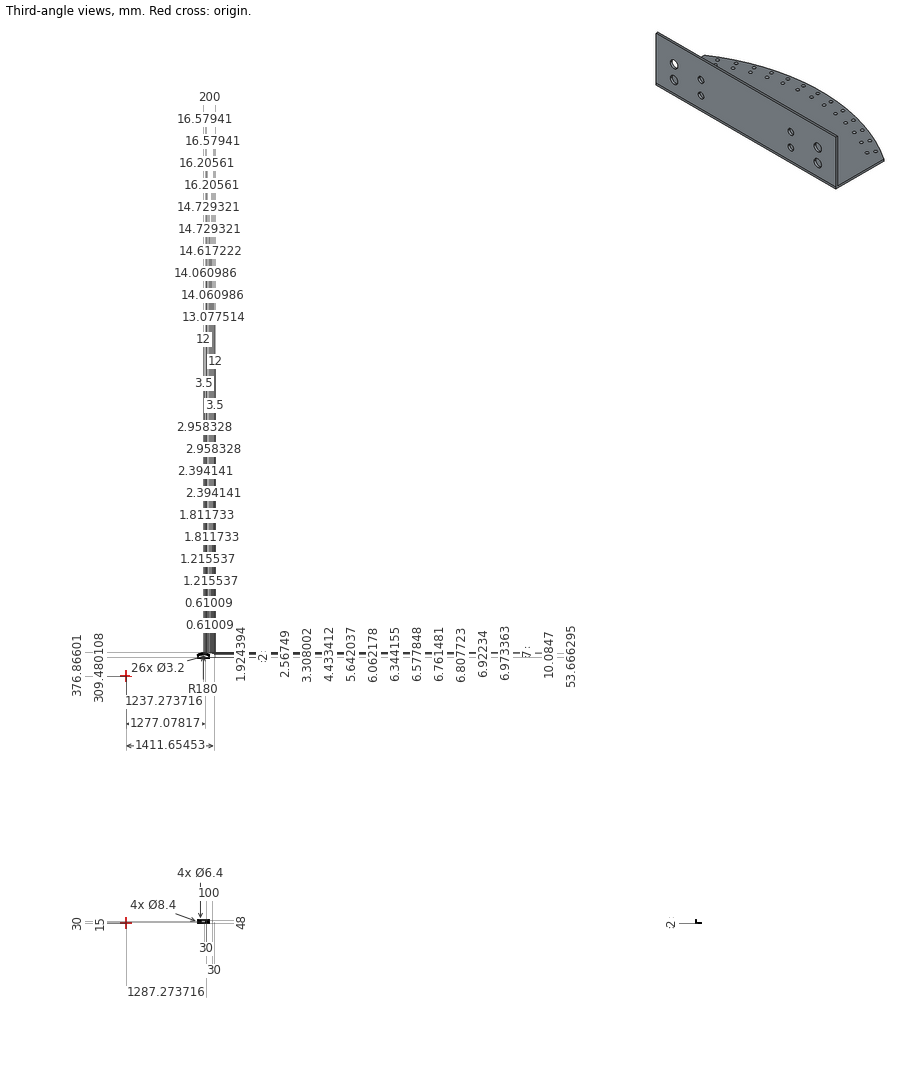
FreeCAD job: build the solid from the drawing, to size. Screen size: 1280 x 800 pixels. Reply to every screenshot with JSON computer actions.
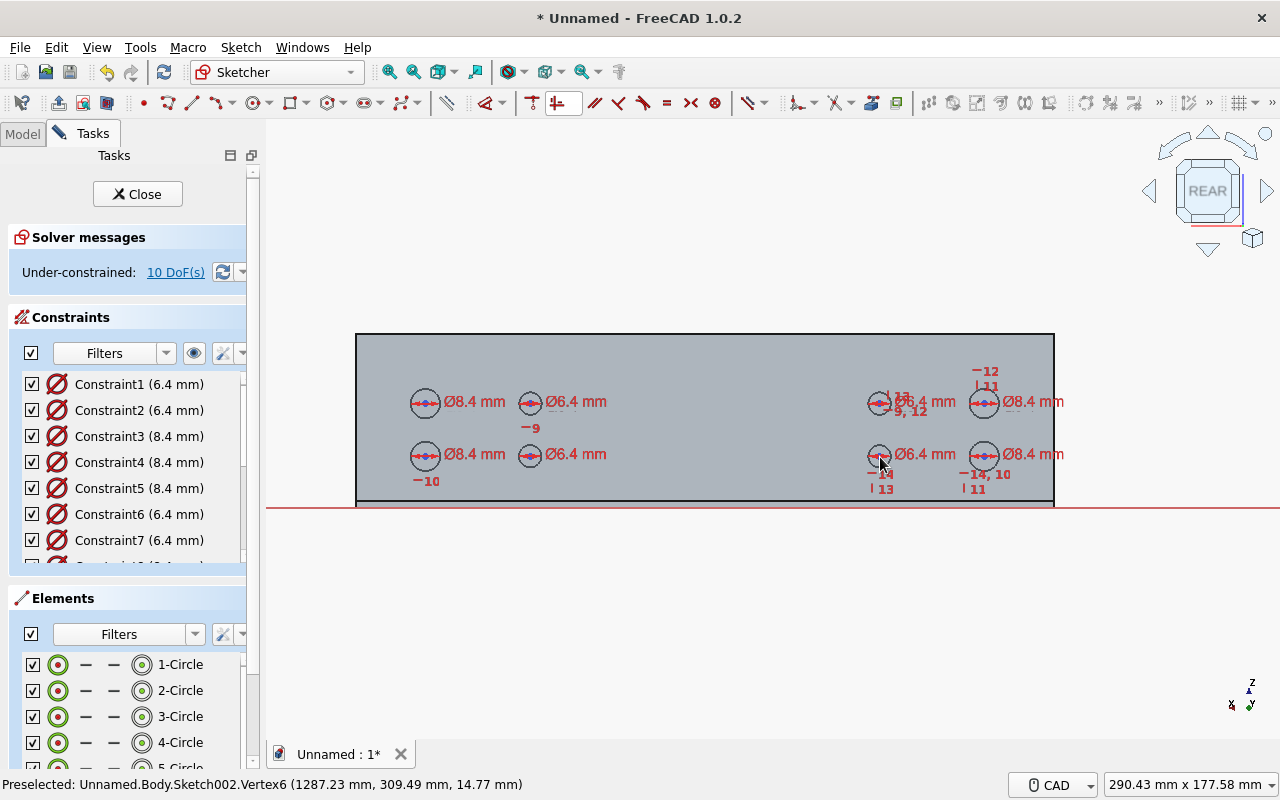
{"action": "left_click", "coordinate": [530, 404]}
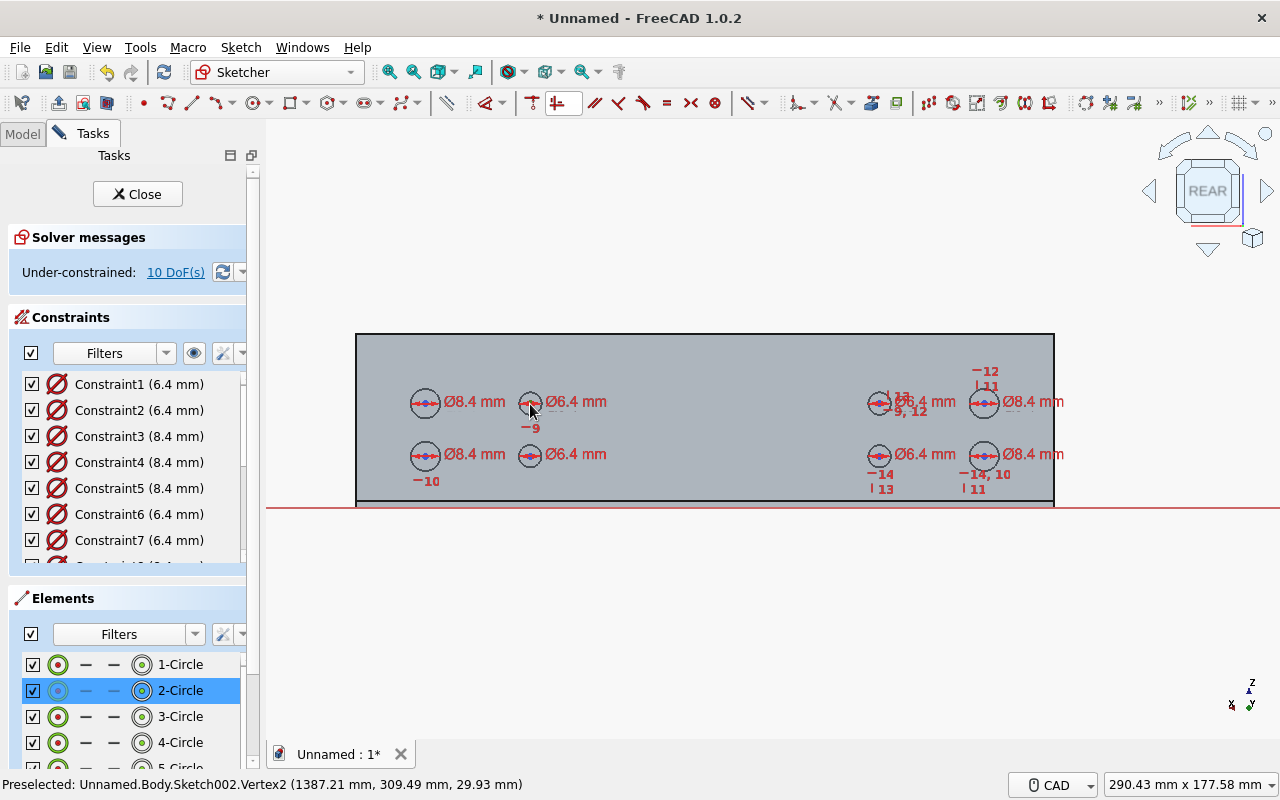
{"action": "left_click", "coordinate": [530, 456]}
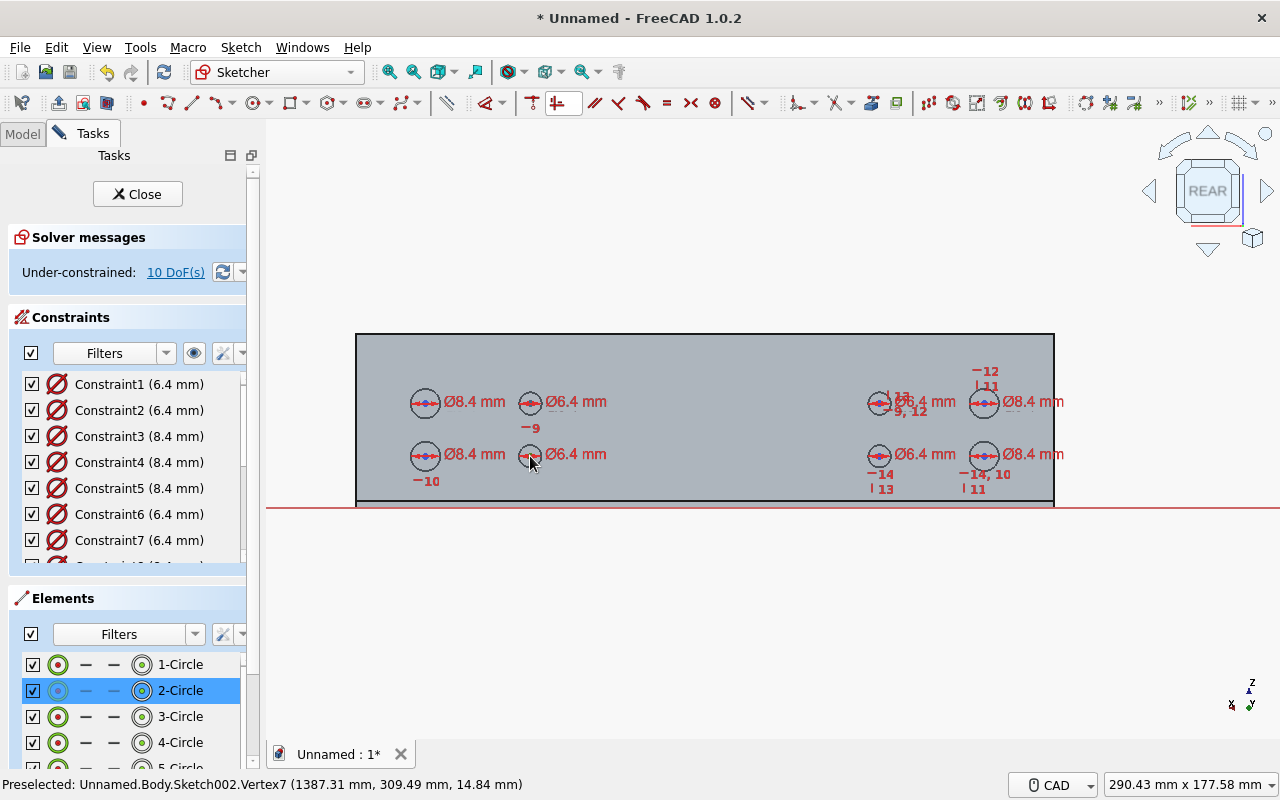
{"action": "key", "text": "v"}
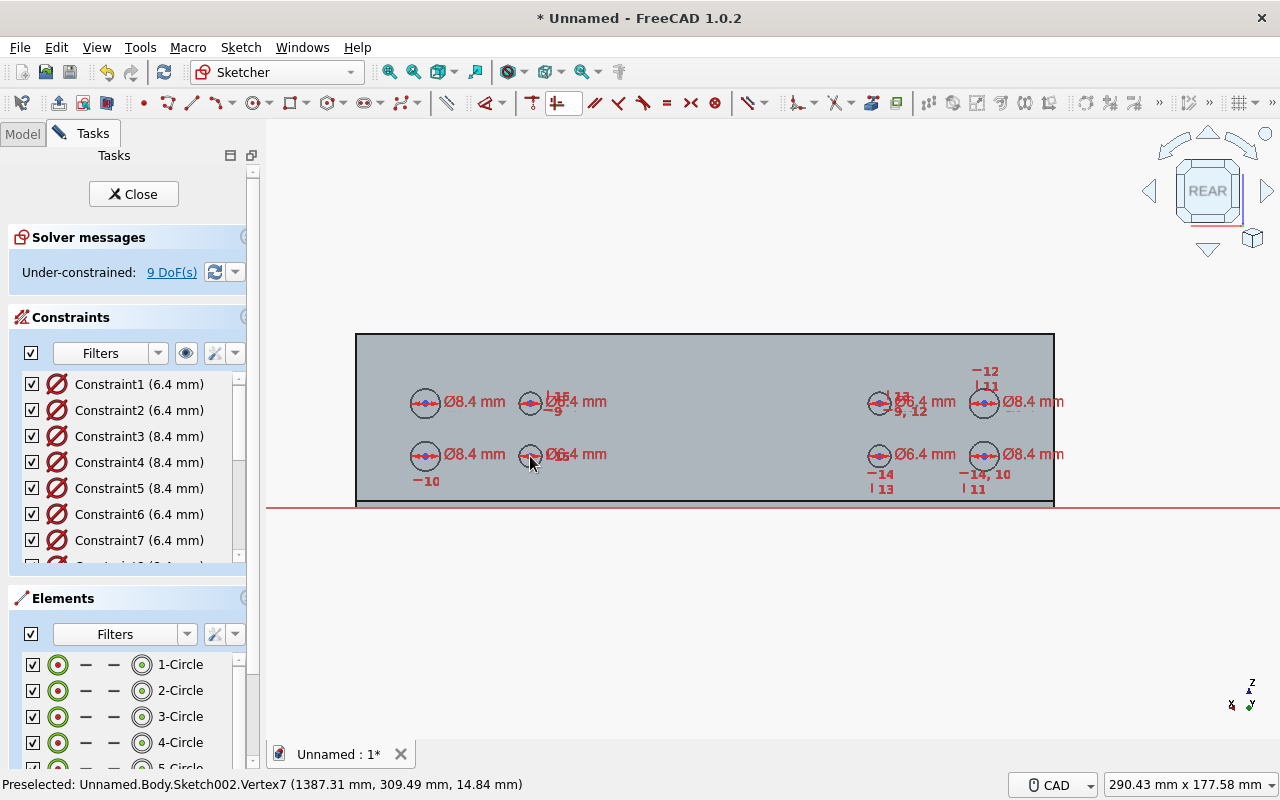
{"action": "left_click", "coordinate": [426, 456]}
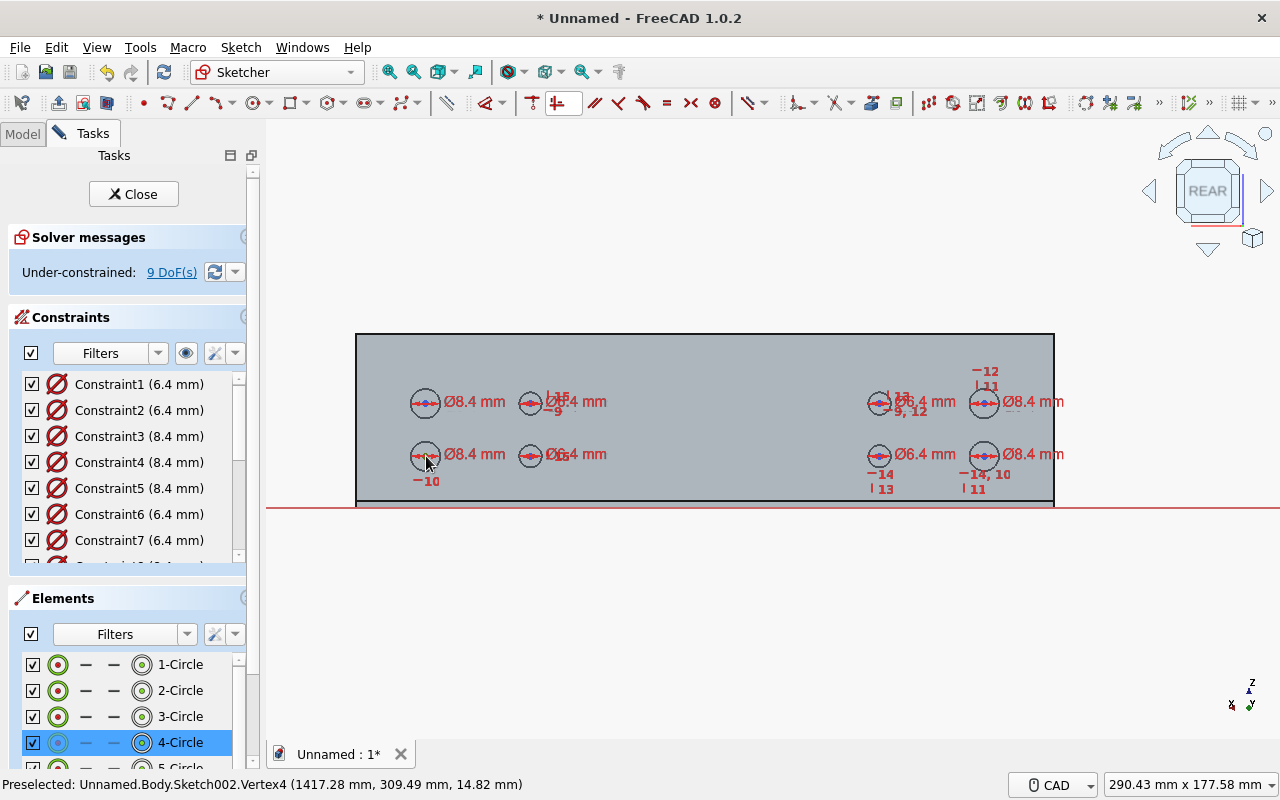
{"action": "left_click", "coordinate": [530, 456]}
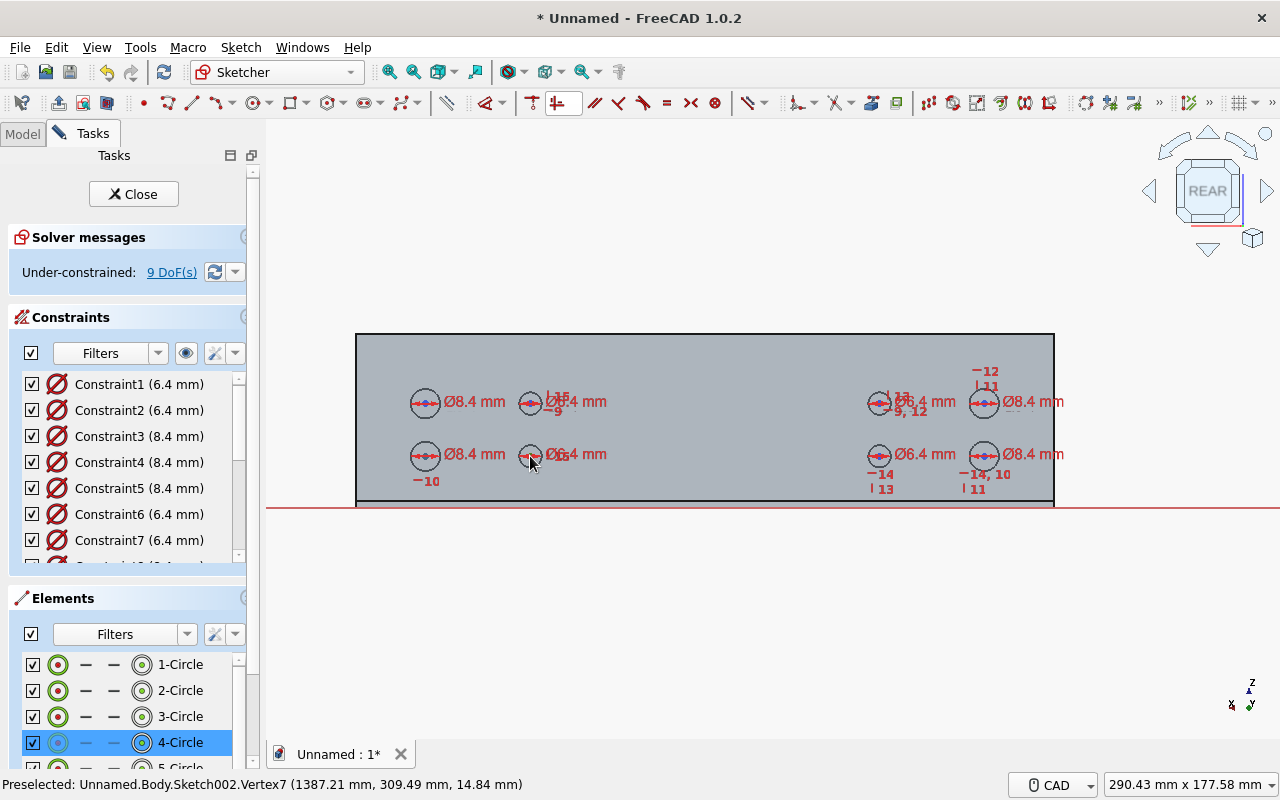
{"action": "key", "text": "h"}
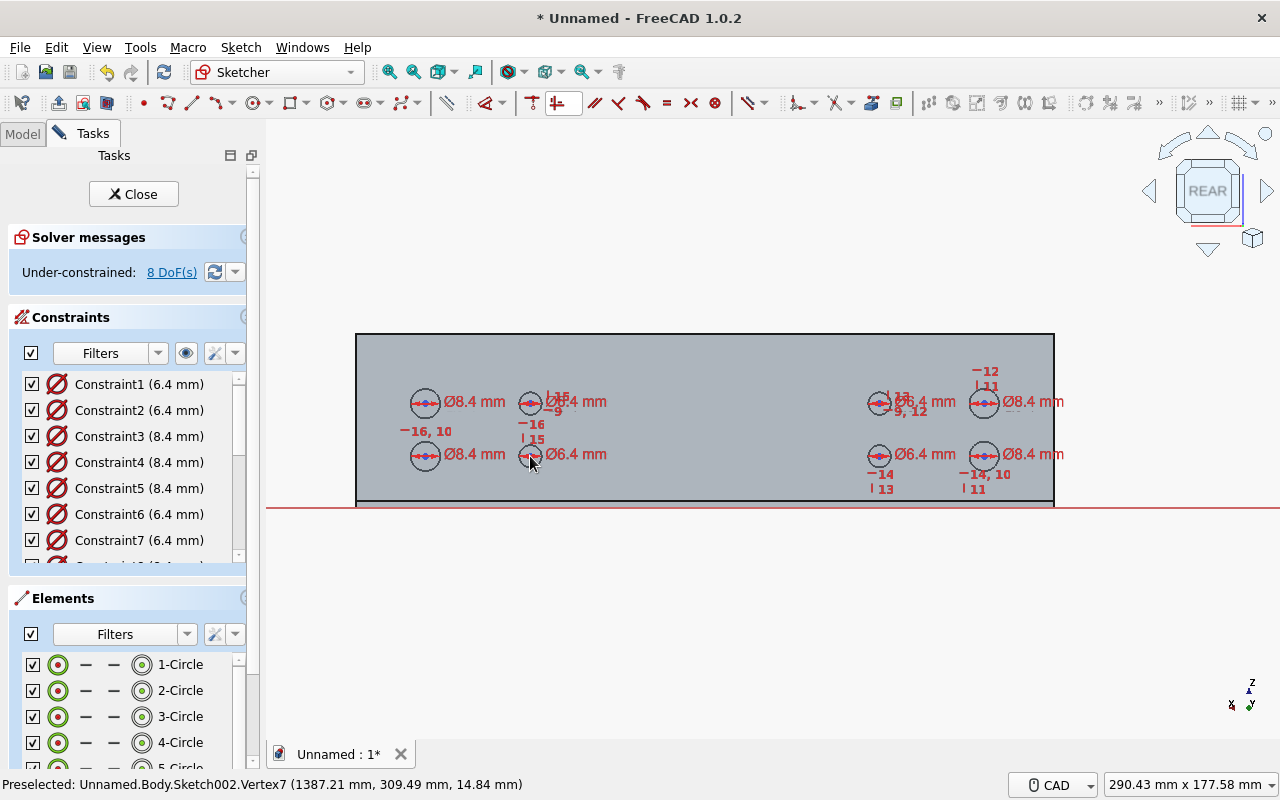
{"action": "left_click", "coordinate": [426, 456]}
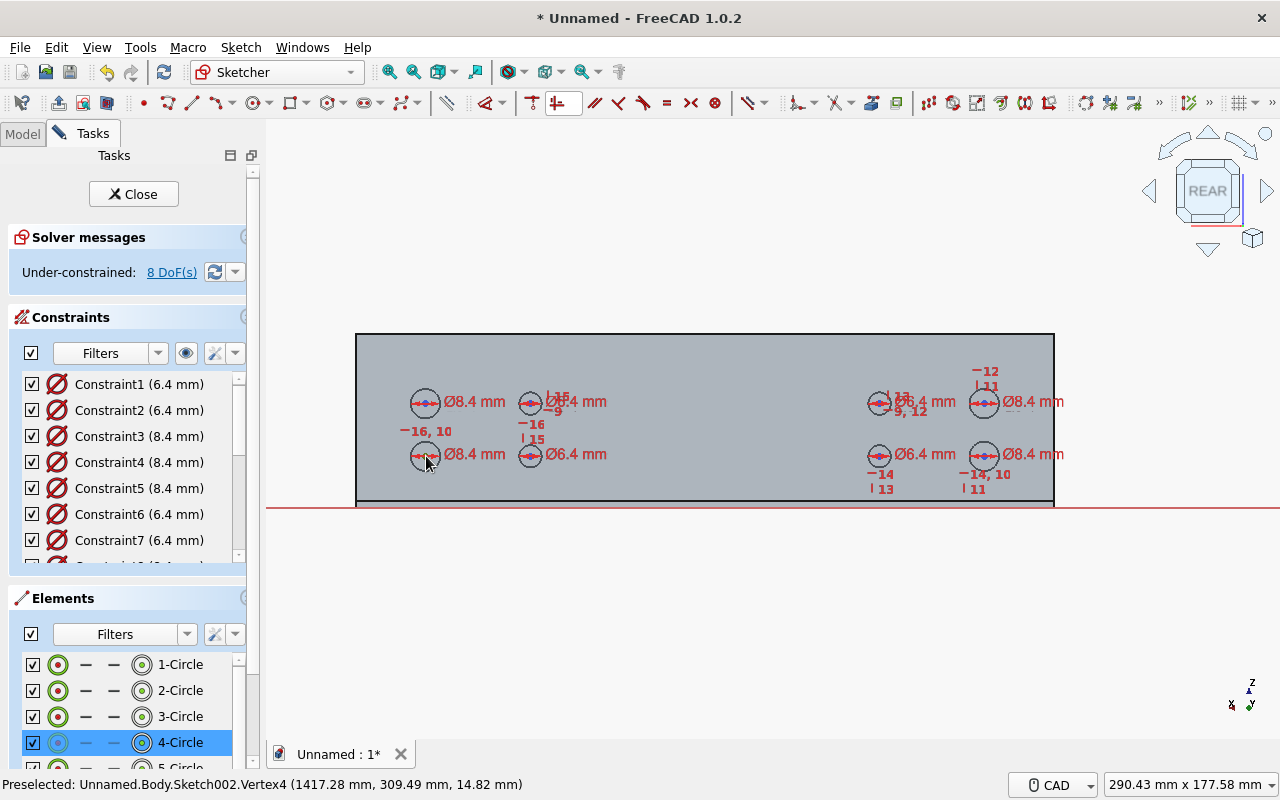
{"action": "left_click", "coordinate": [425, 404]}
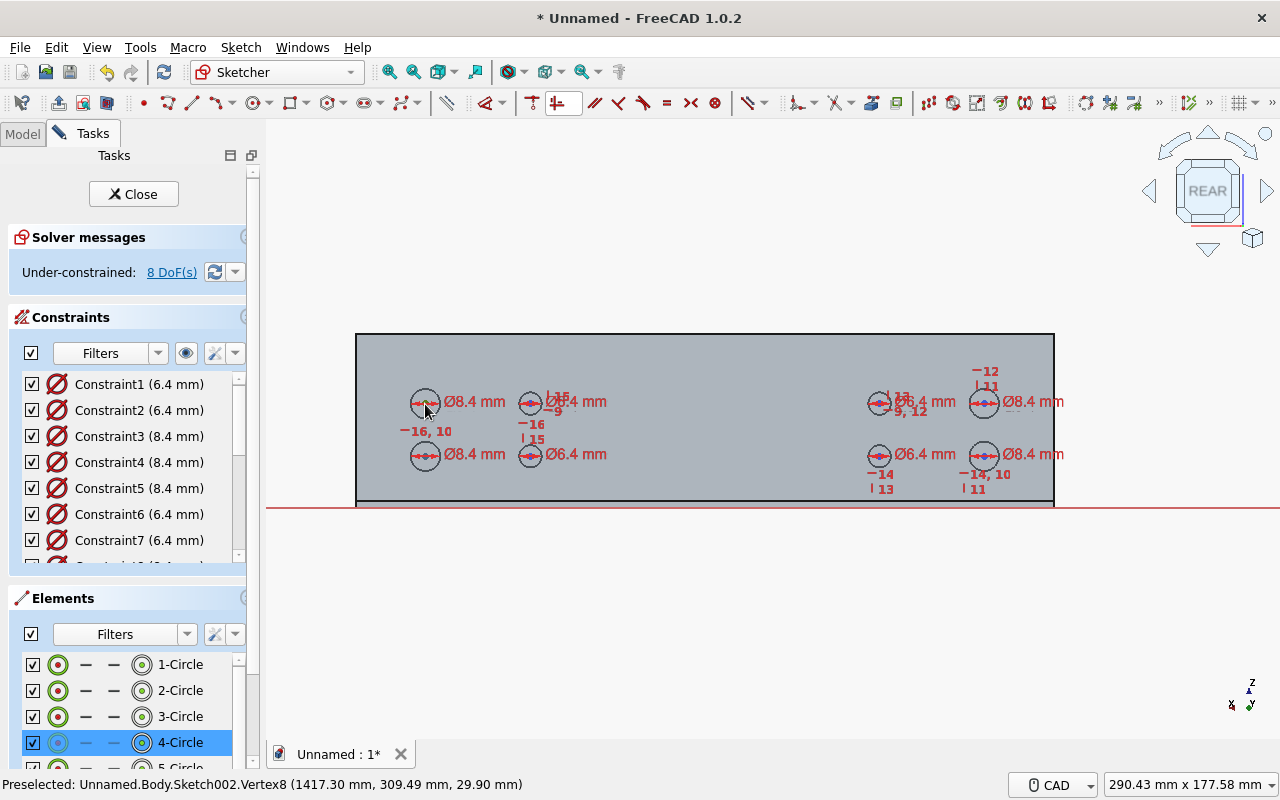
{"action": "key", "text": "v"}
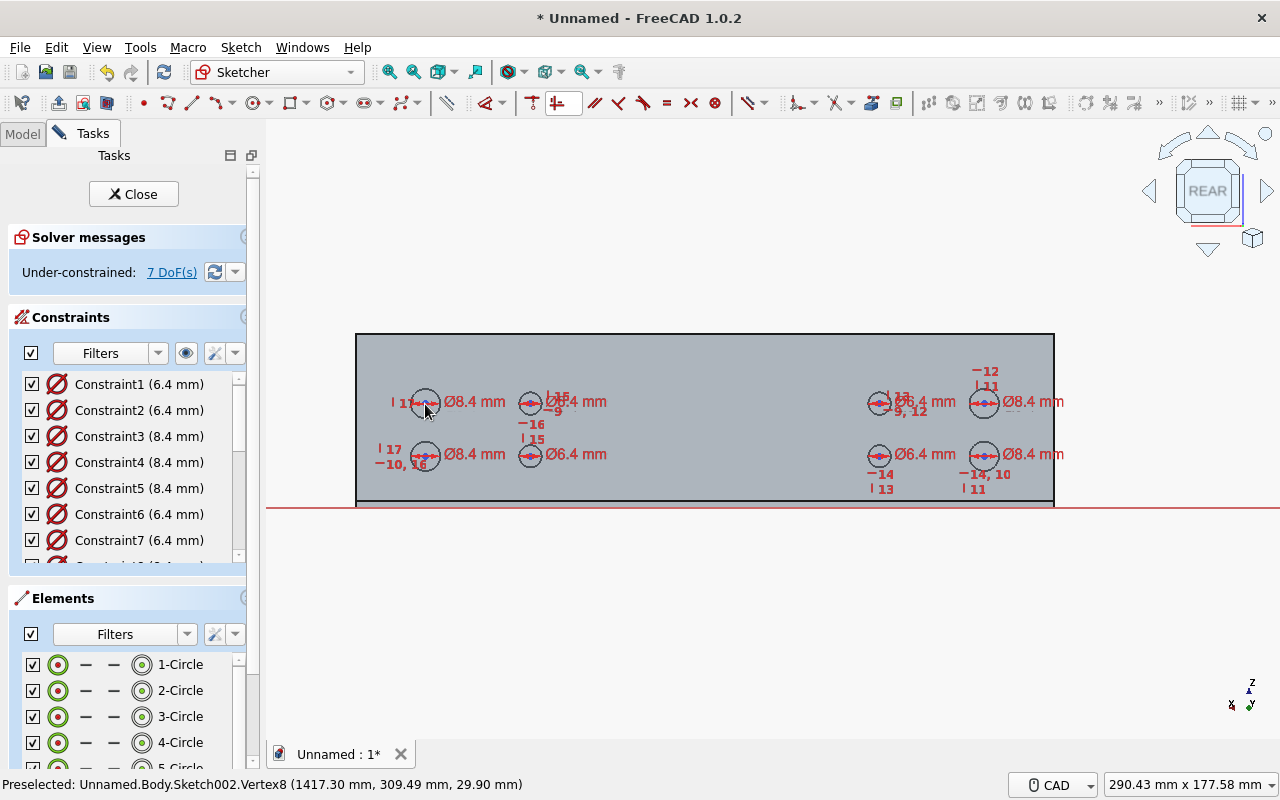
{"action": "left_click", "coordinate": [530, 404]}